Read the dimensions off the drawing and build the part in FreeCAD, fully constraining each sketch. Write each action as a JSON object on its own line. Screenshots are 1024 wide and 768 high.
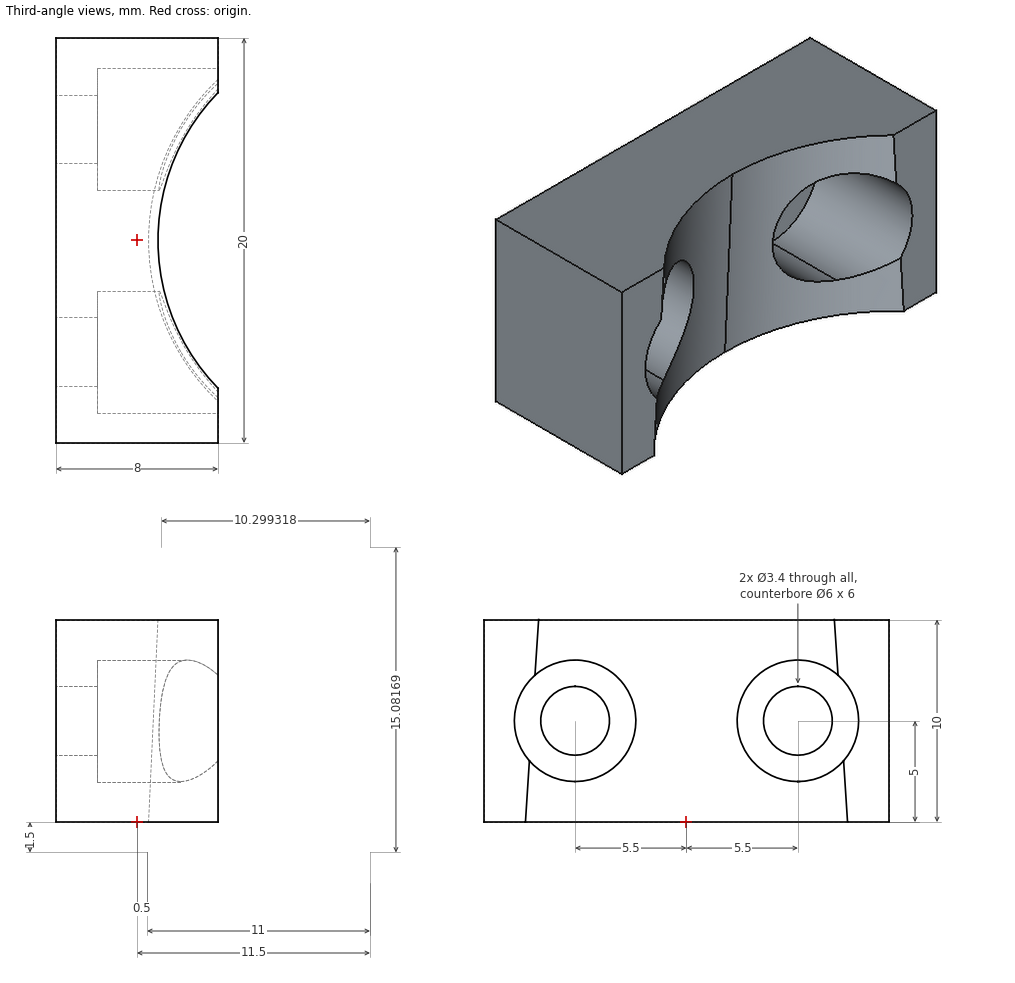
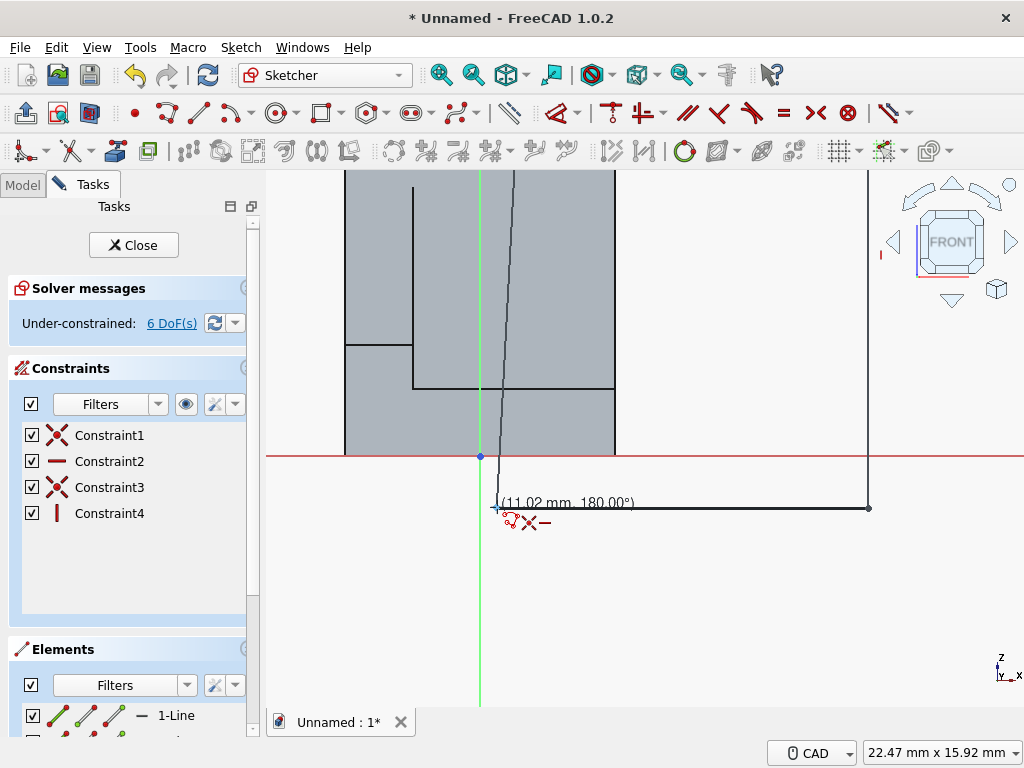
{"action": "left_click", "coordinate": [497, 508]}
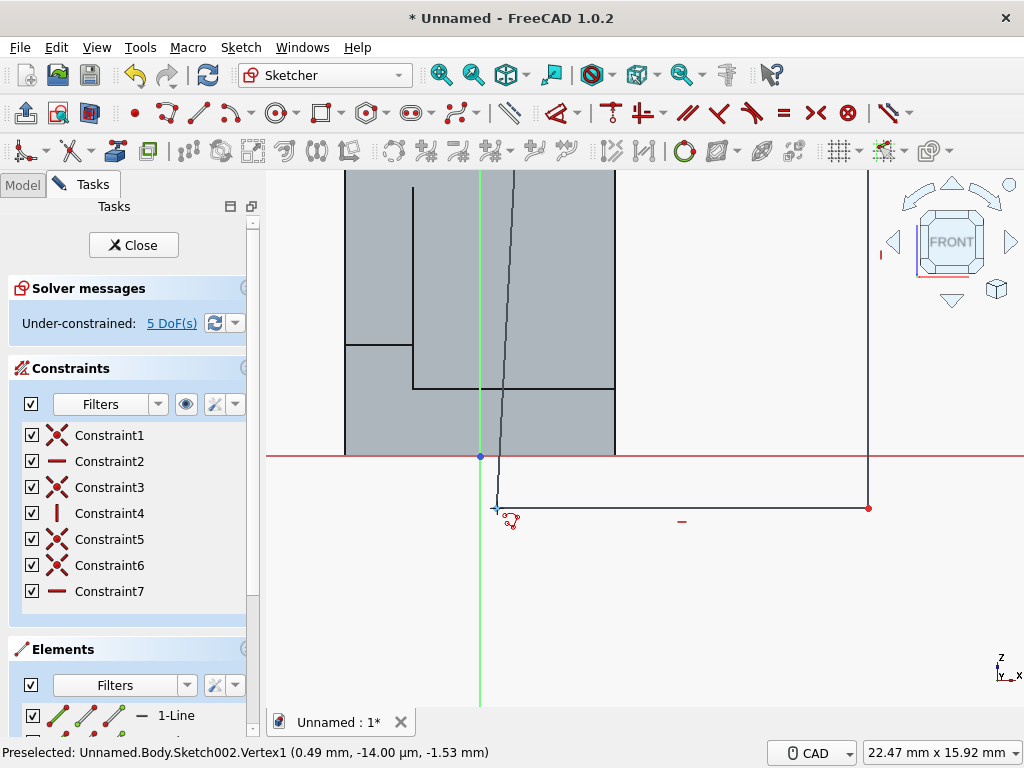
{"action": "key", "text": "g l"}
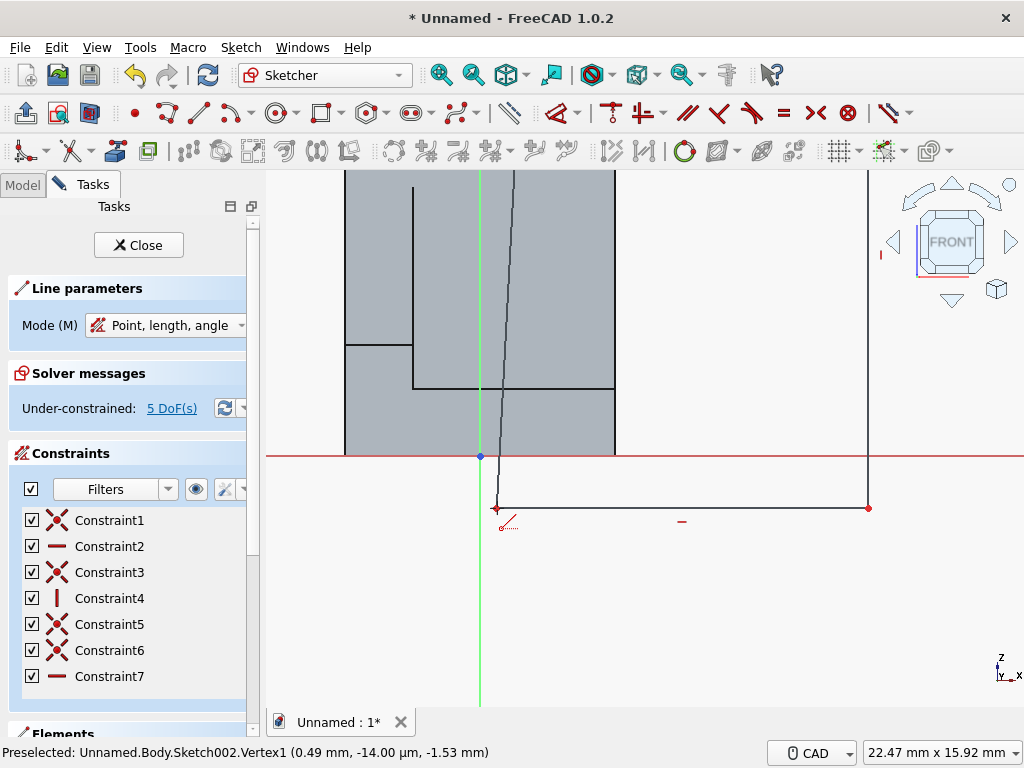
{"action": "scroll", "coordinate": [497, 507], "scroll_direction": "down", "scroll_amount": 4}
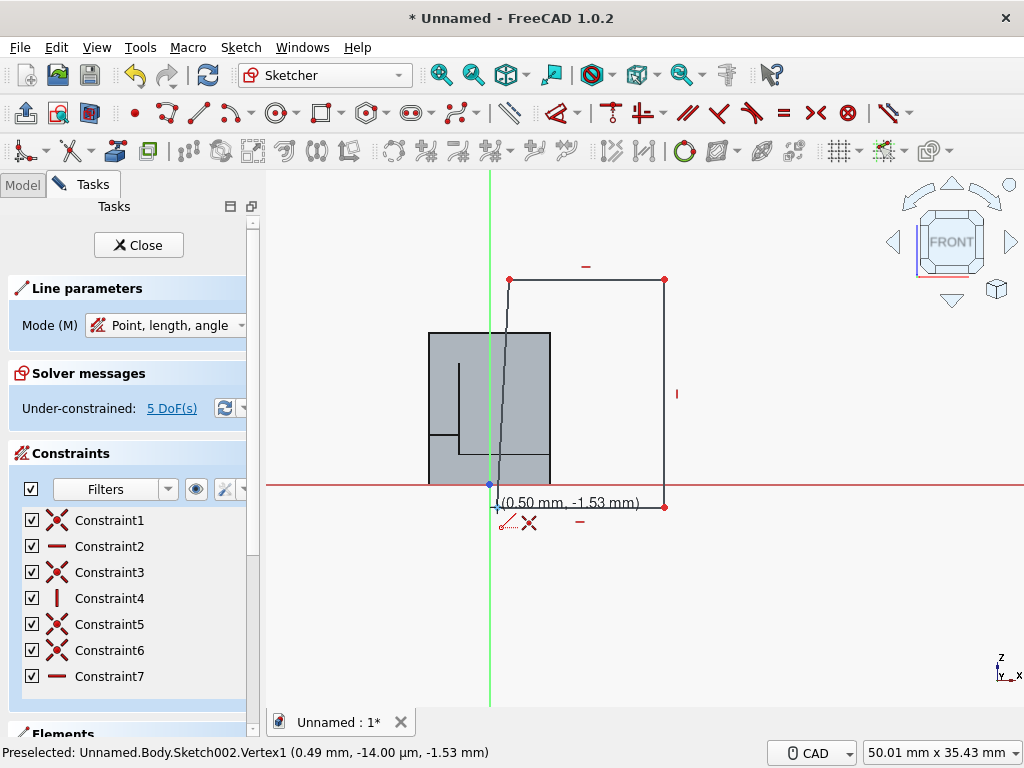
{"action": "left_click", "coordinate": [664, 530]}
{"action": "left_click", "coordinate": [664, 599]}
{"action": "key", "text": "Escape"}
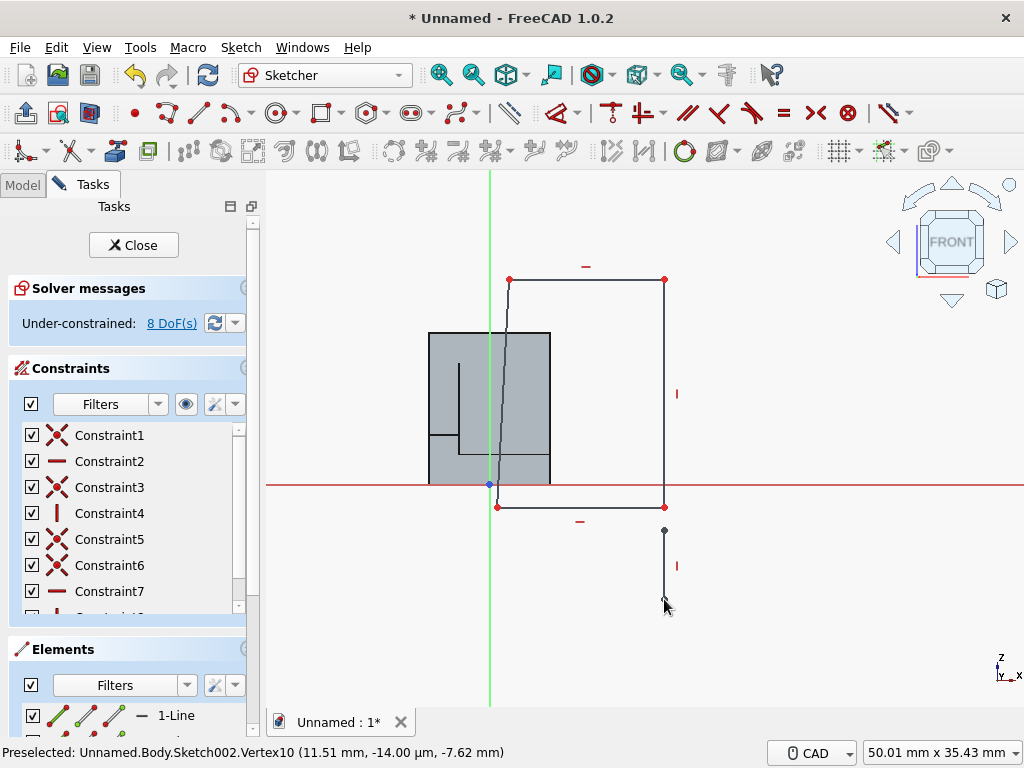
{"action": "left_click", "coordinate": [664, 552]}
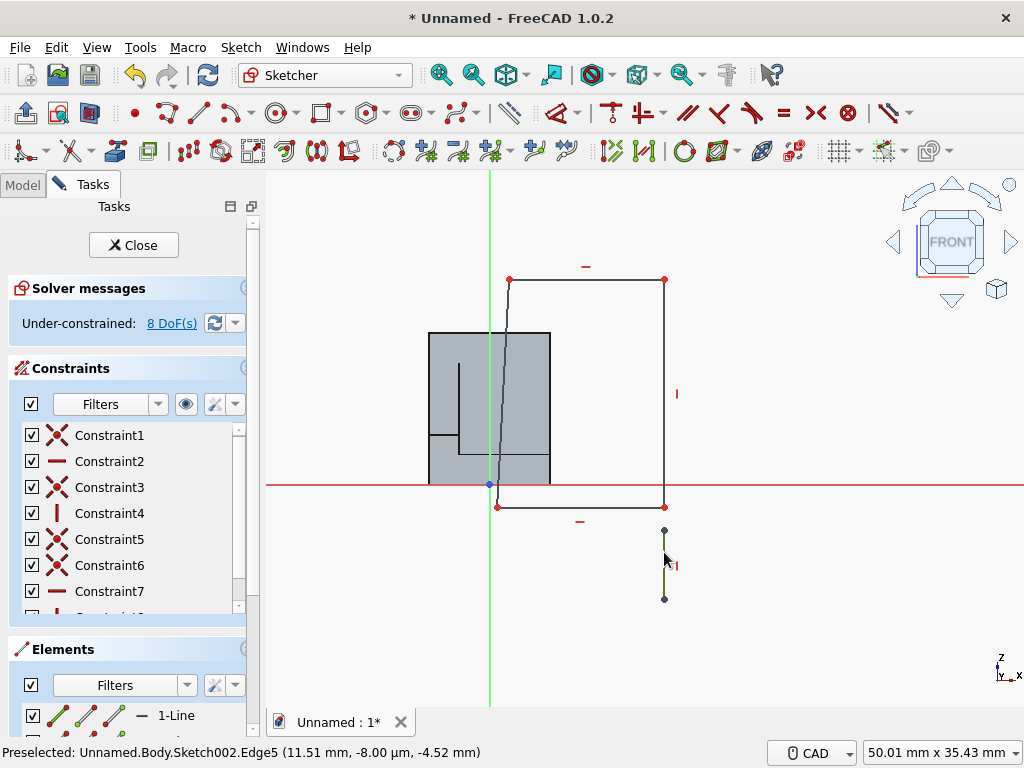
{"action": "key", "text": "g n"}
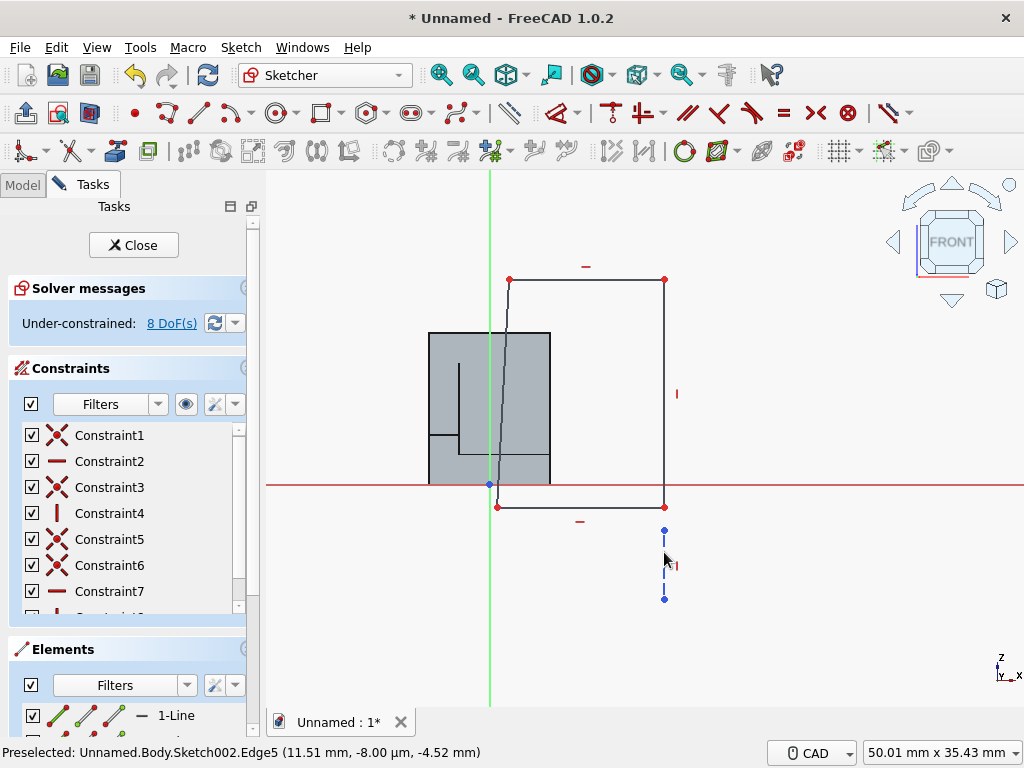
{"action": "left_click", "coordinate": [556, 114]}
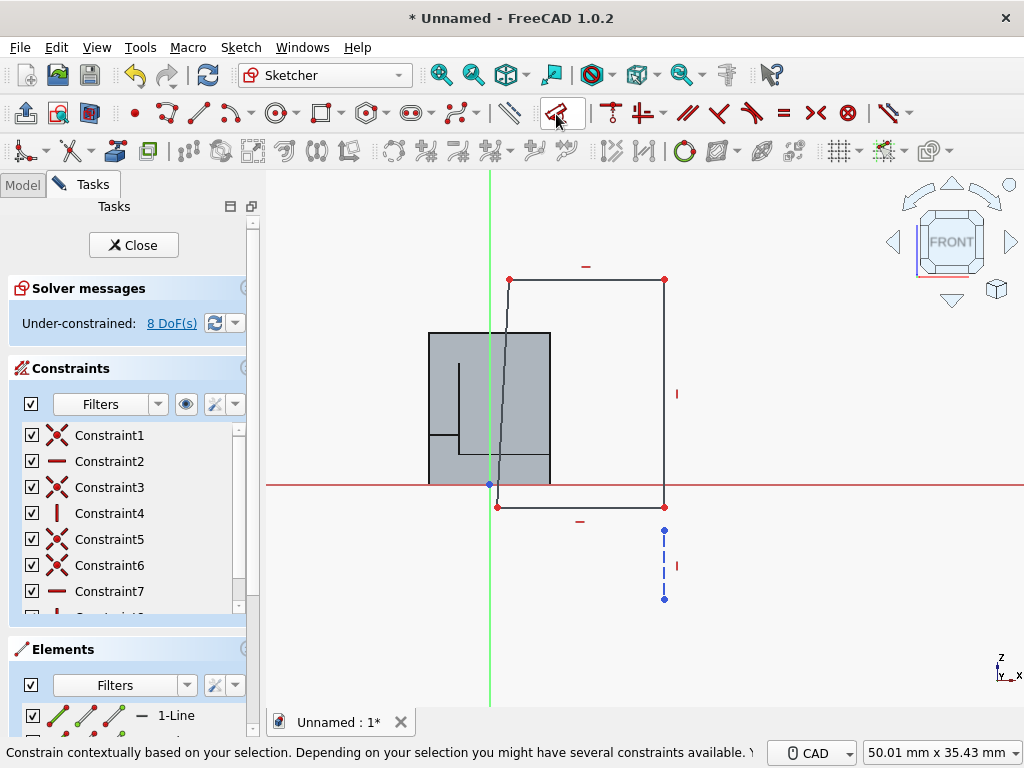
{"action": "left_click", "coordinate": [614, 508]}
{"action": "left_click", "coordinate": [581, 542]}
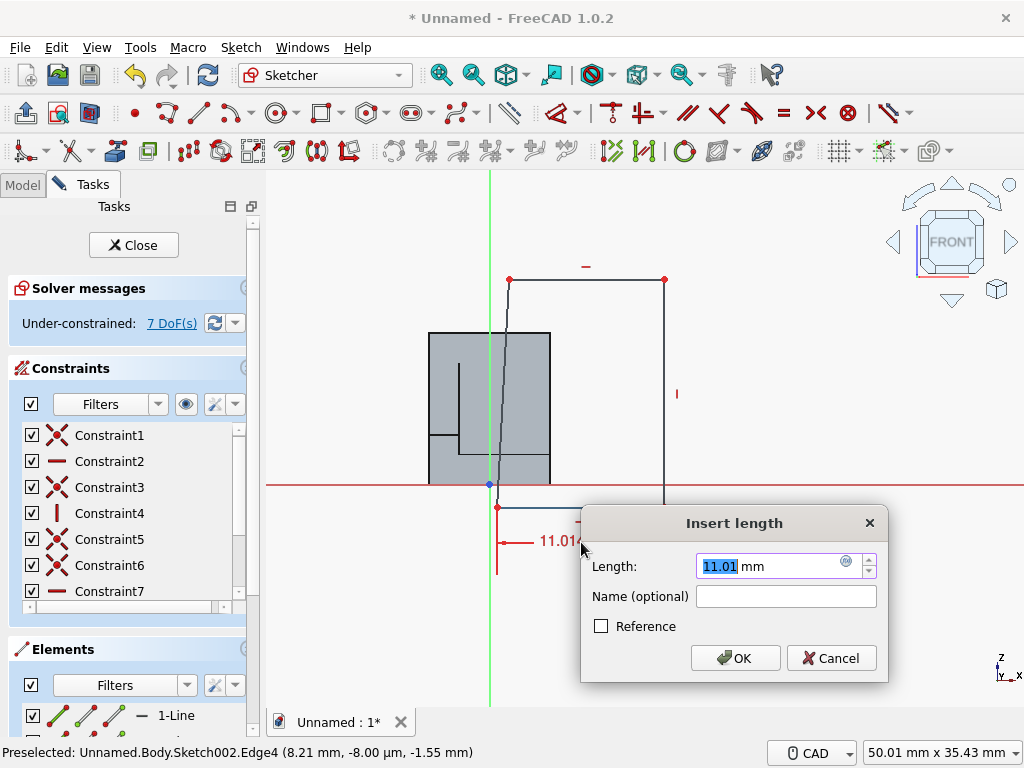
{"action": "type", "text": "11"}
{"action": "key", "text": "Return"}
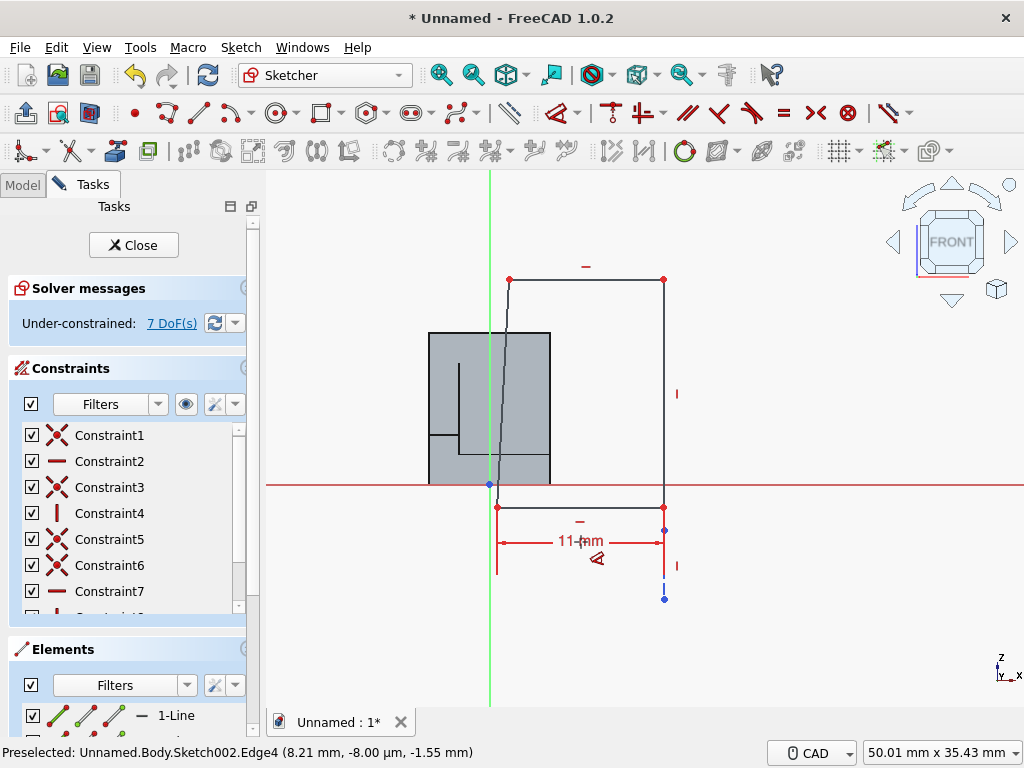
{"action": "scroll", "coordinate": [497, 508], "scroll_direction": "up", "scroll_amount": 9}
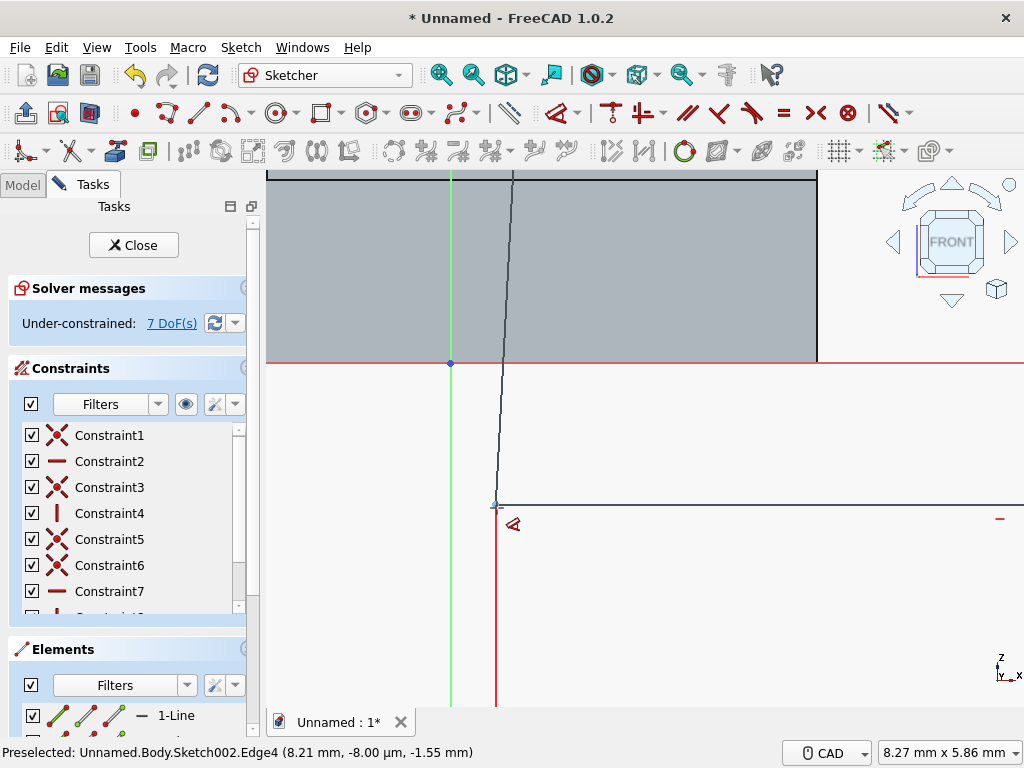
{"action": "left_click", "coordinate": [496, 505]}
{"action": "left_click", "coordinate": [473, 539]}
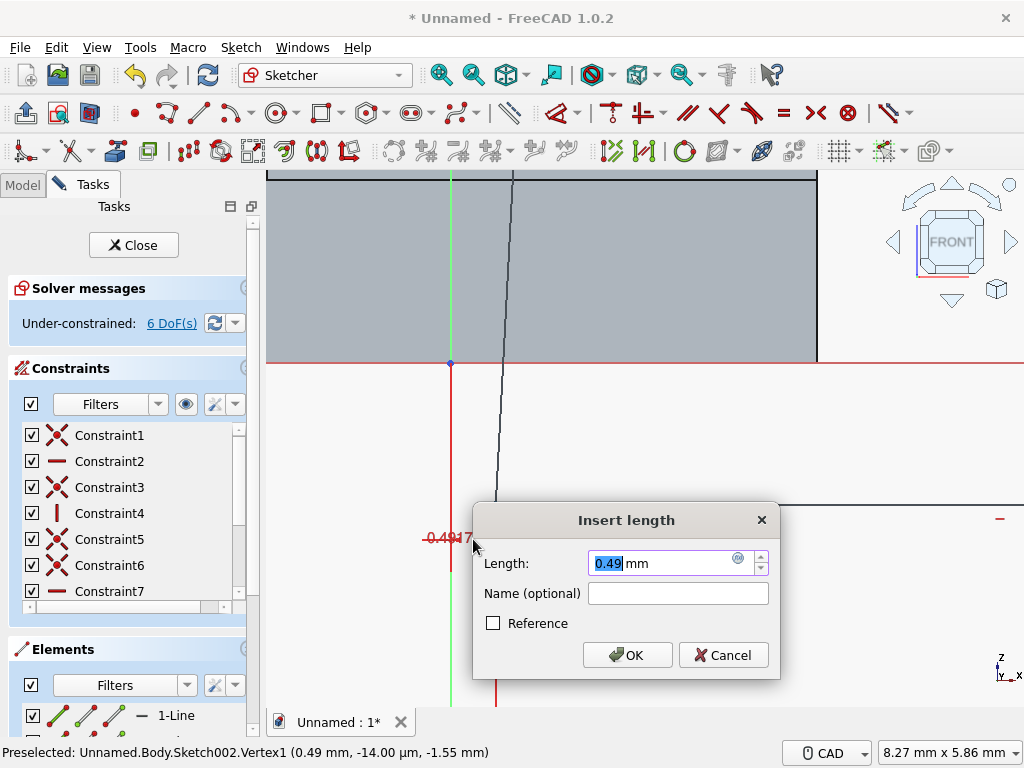
{"action": "type", "text": "0.5"}
{"action": "key", "text": "Return"}